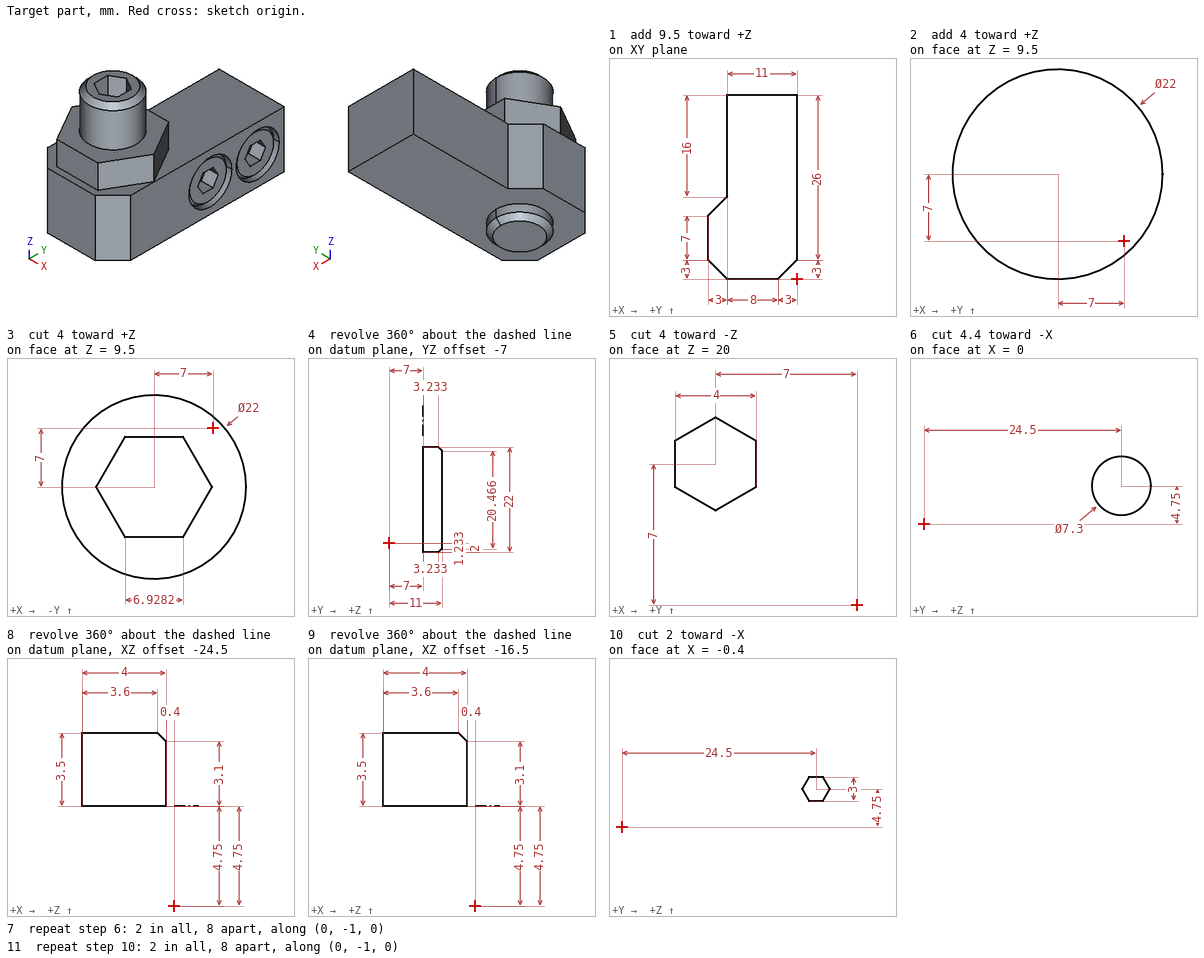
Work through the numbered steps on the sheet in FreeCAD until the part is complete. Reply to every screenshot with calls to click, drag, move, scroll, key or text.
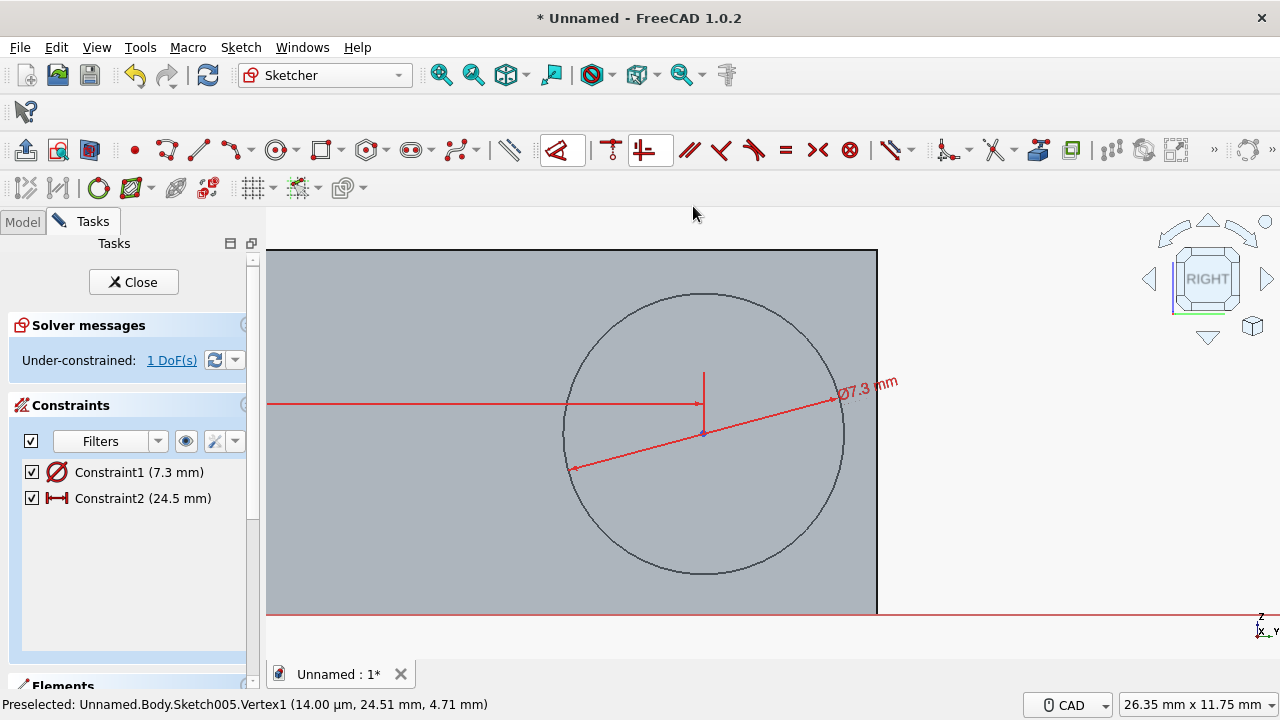
click(704, 434)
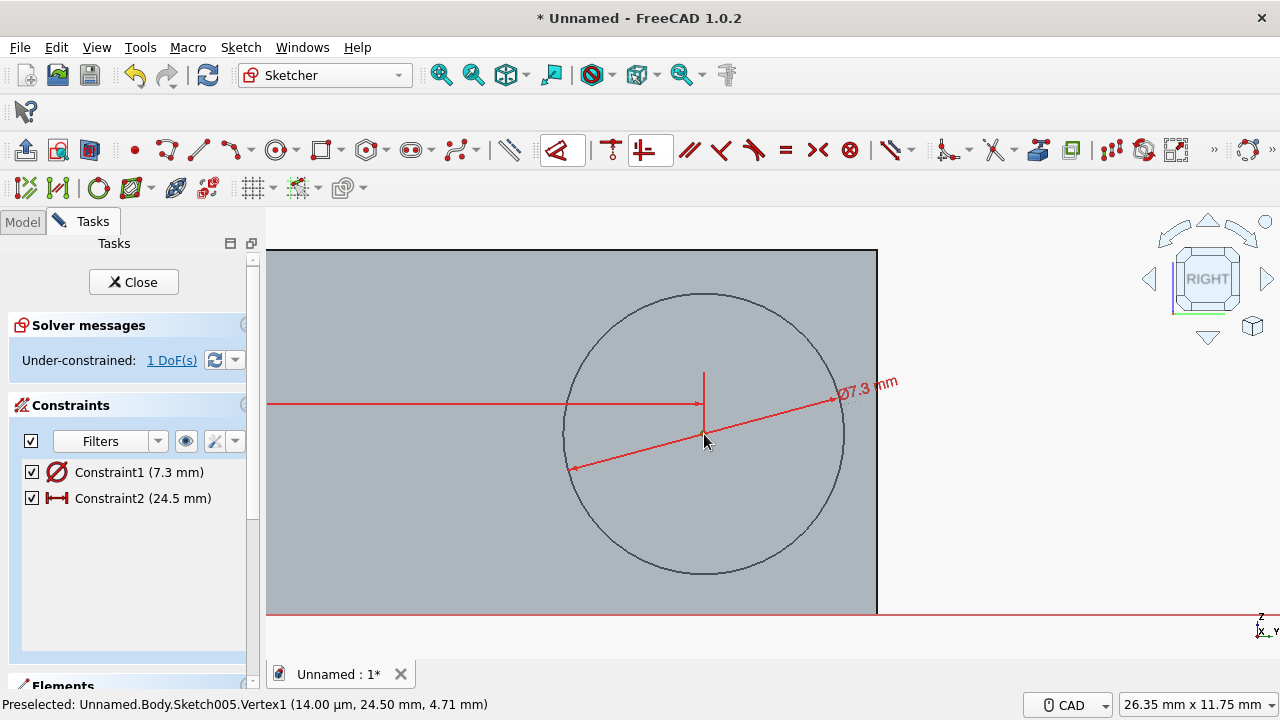
key(i)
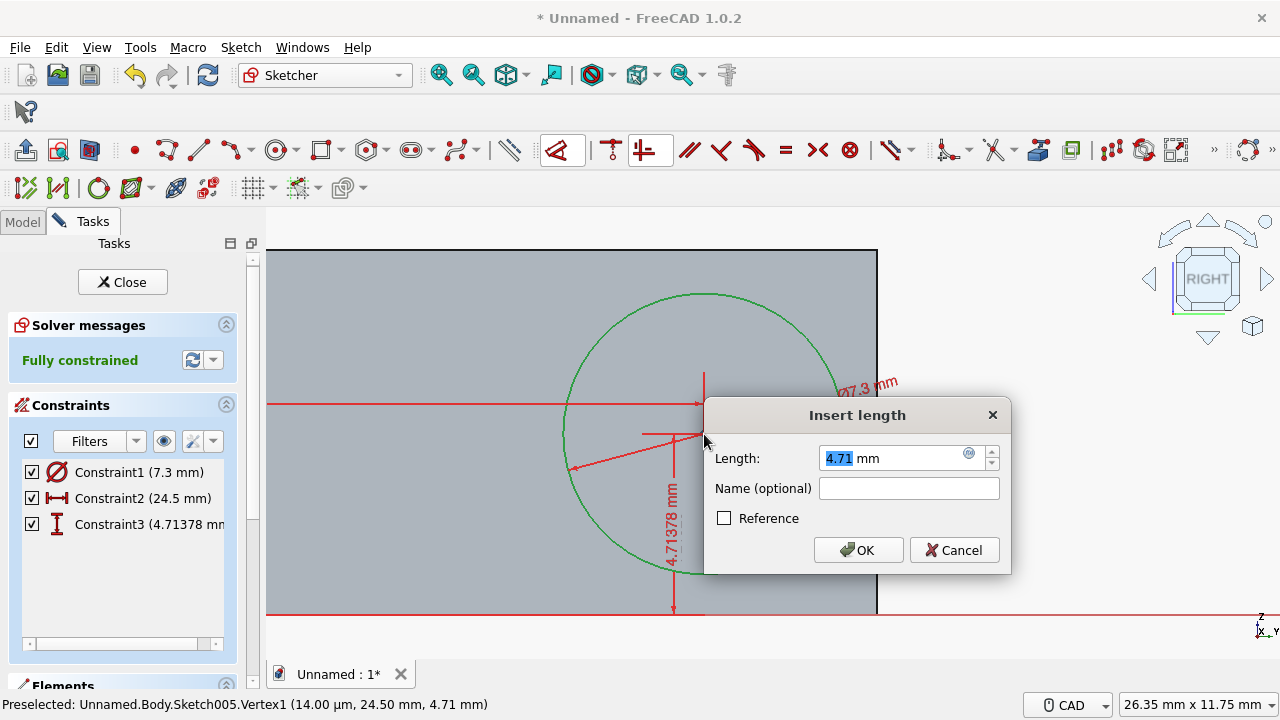
text(4.75)
key(Return)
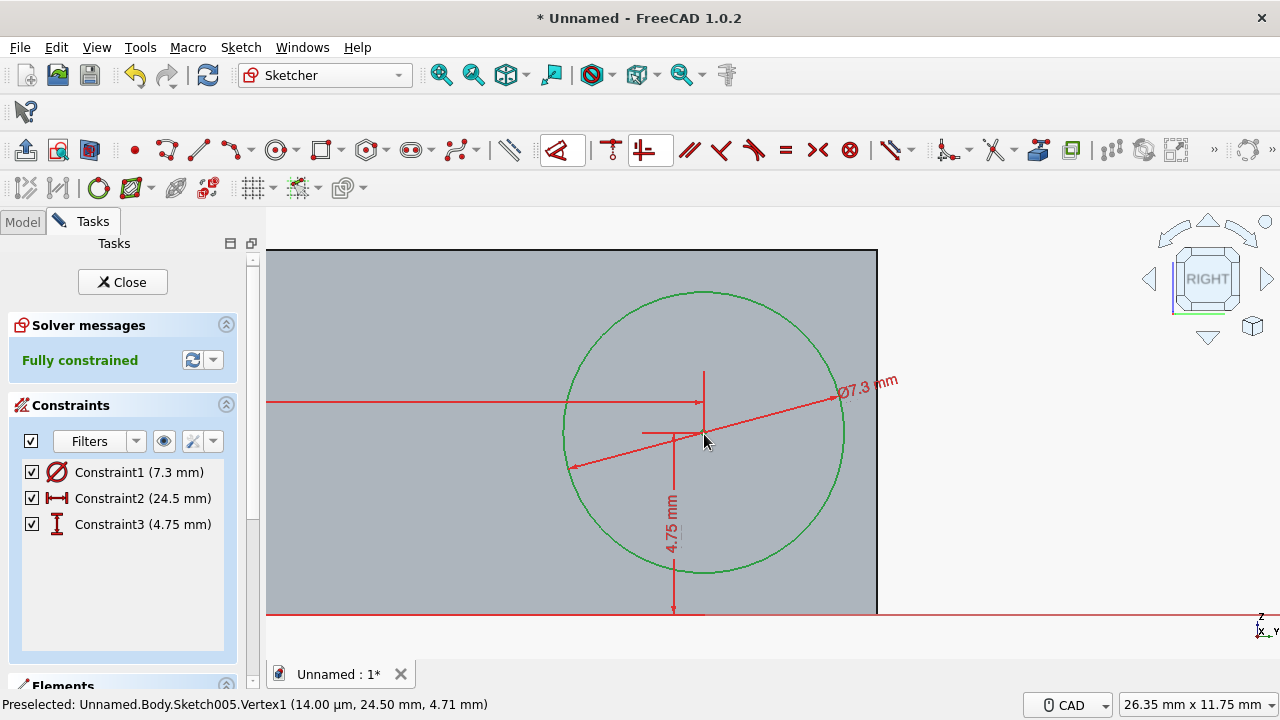
click(123, 282)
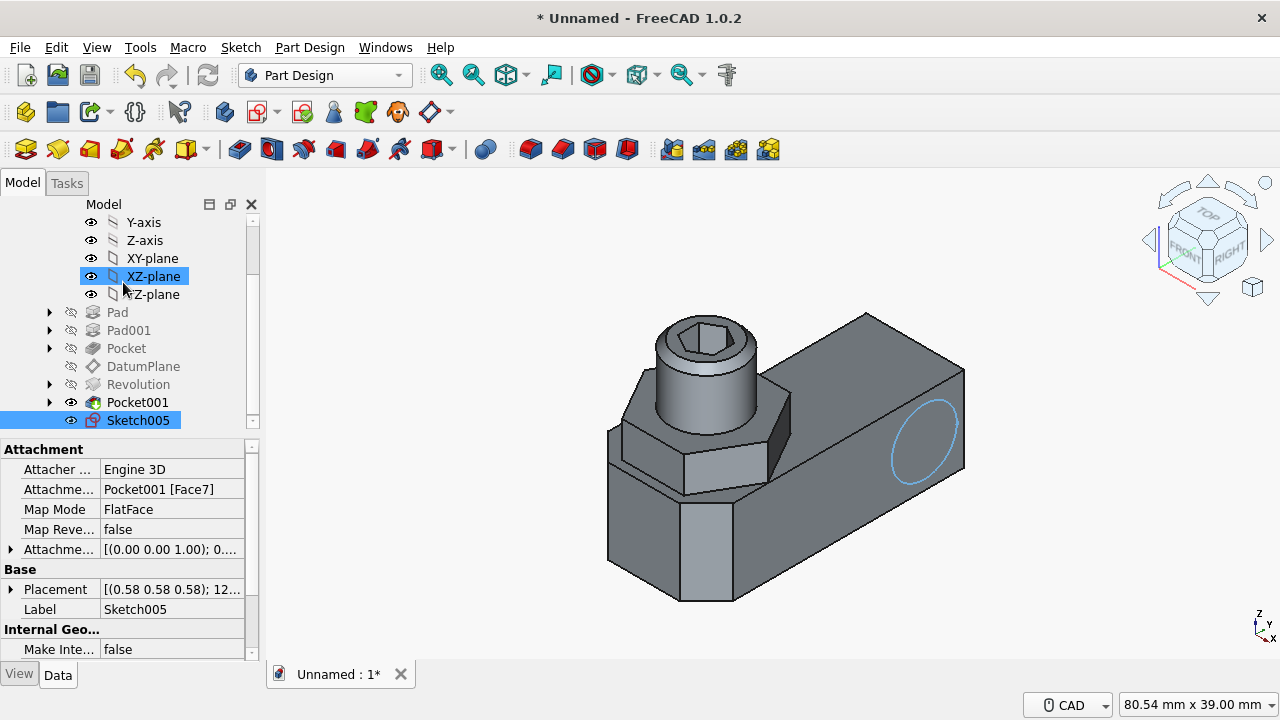
click(240, 150)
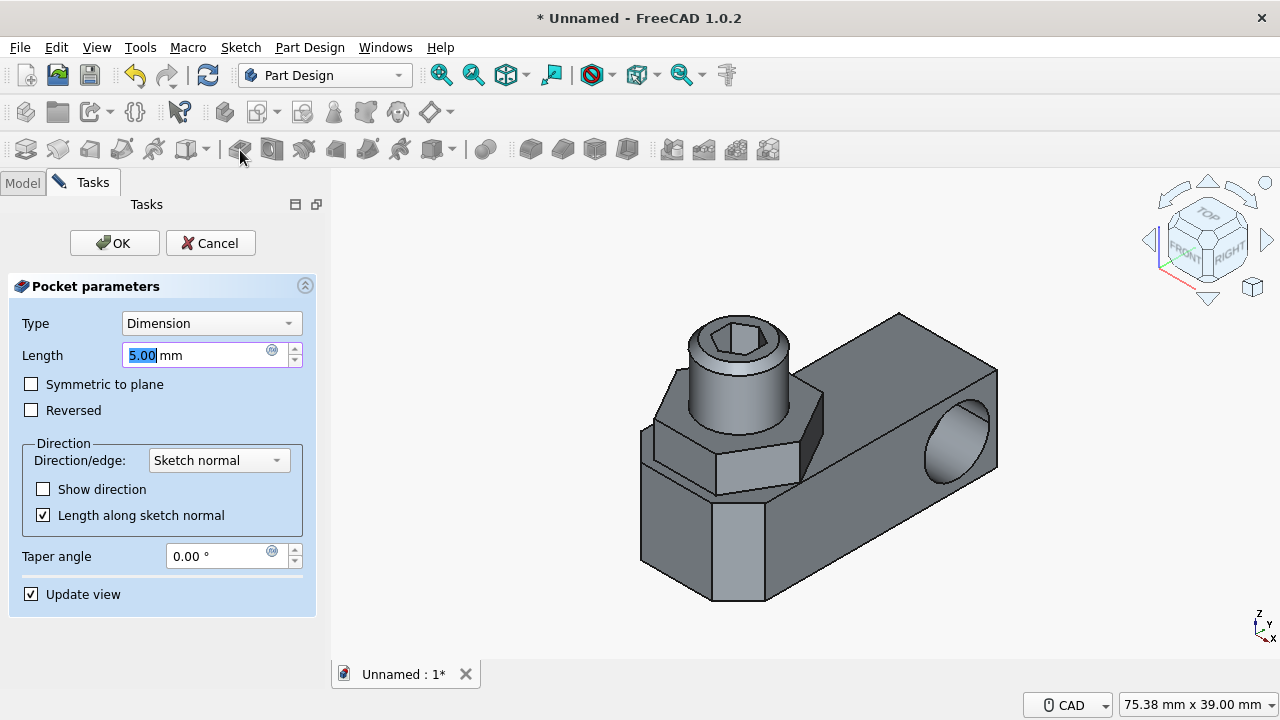
text(4.4)
key(Tab)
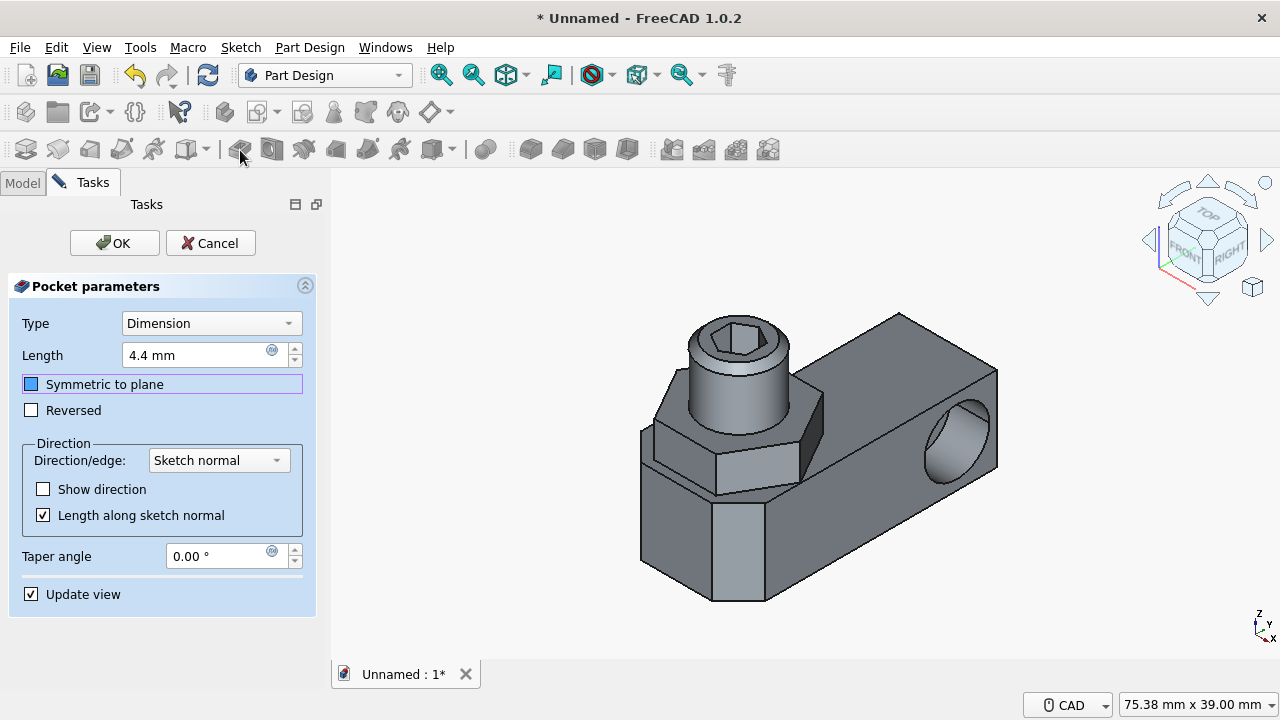
click(115, 243)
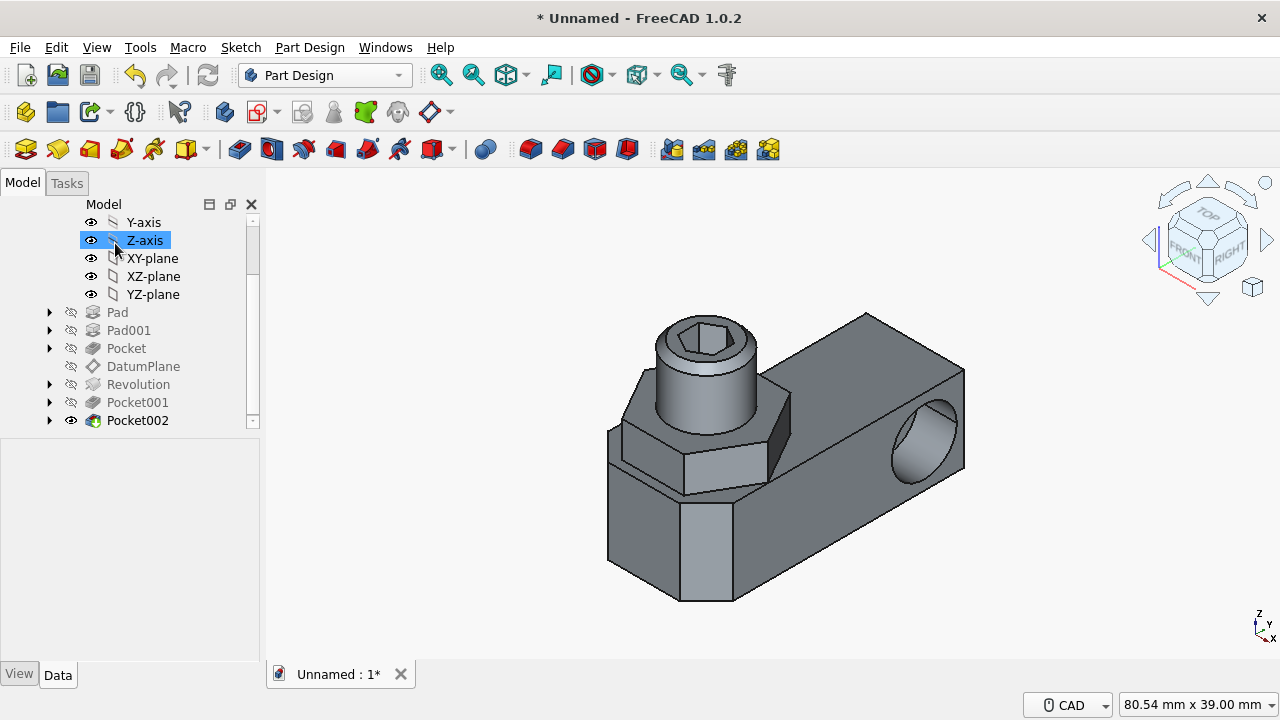
click(116, 420)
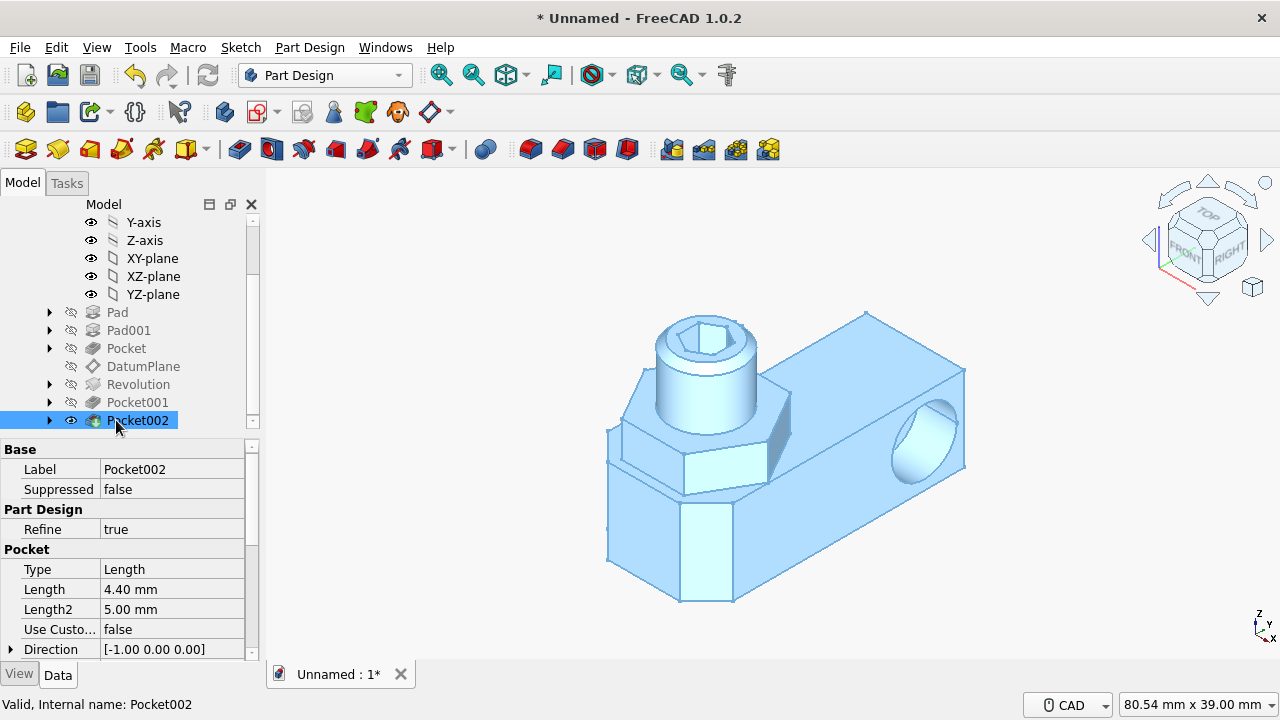
click(704, 150)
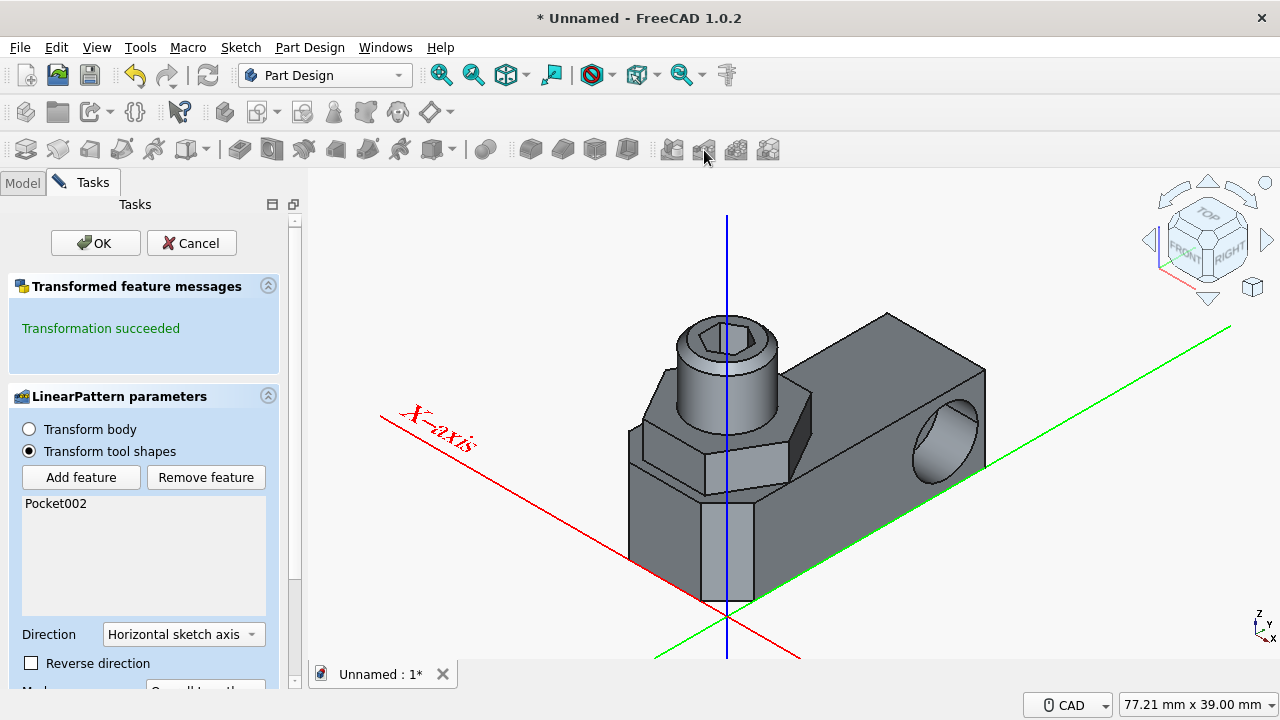
click(184, 634)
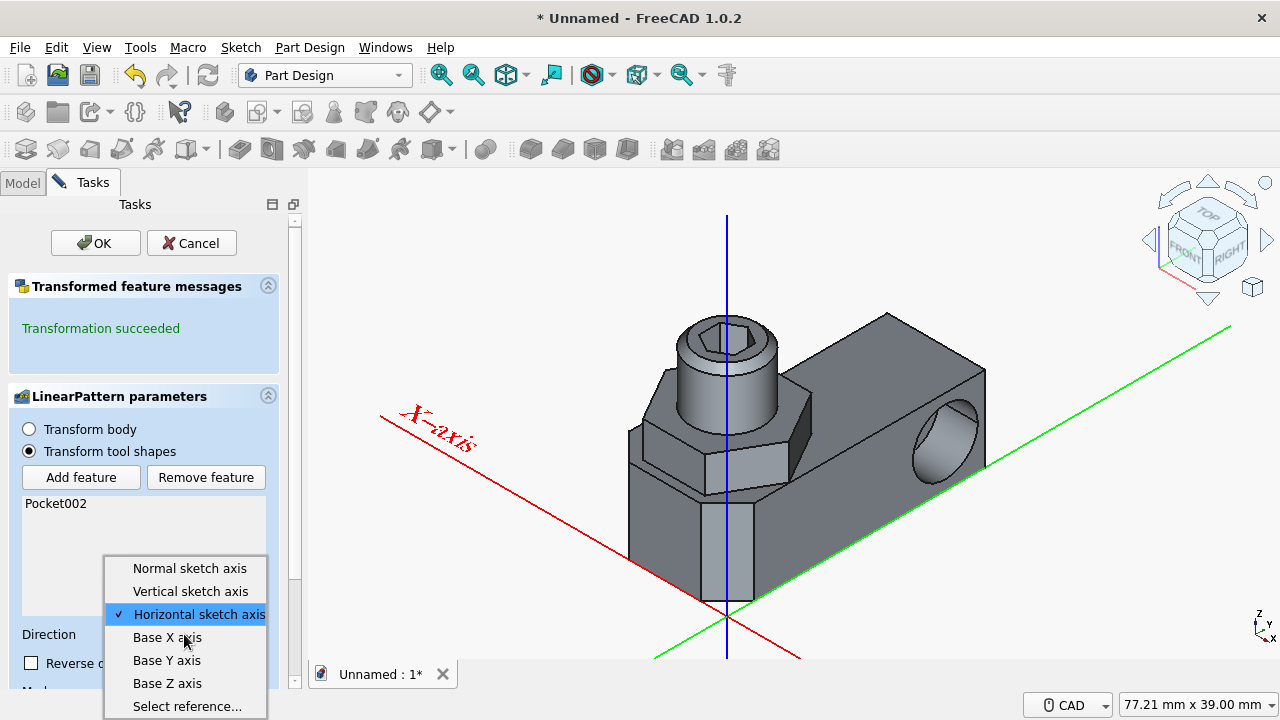
click(184, 660)